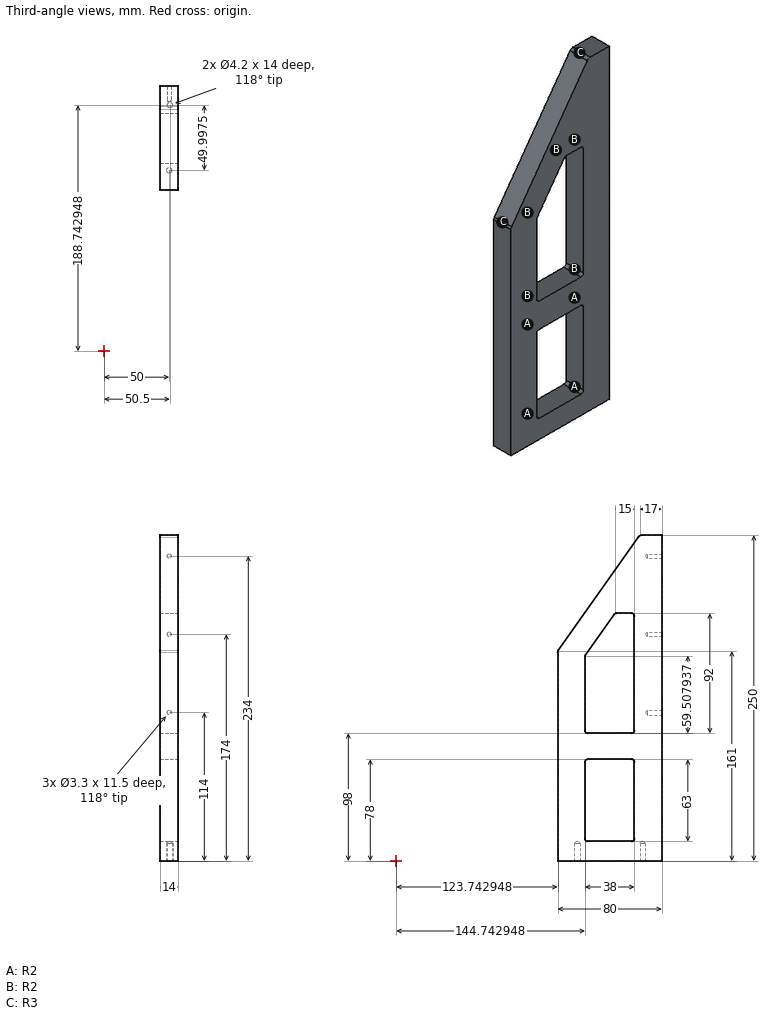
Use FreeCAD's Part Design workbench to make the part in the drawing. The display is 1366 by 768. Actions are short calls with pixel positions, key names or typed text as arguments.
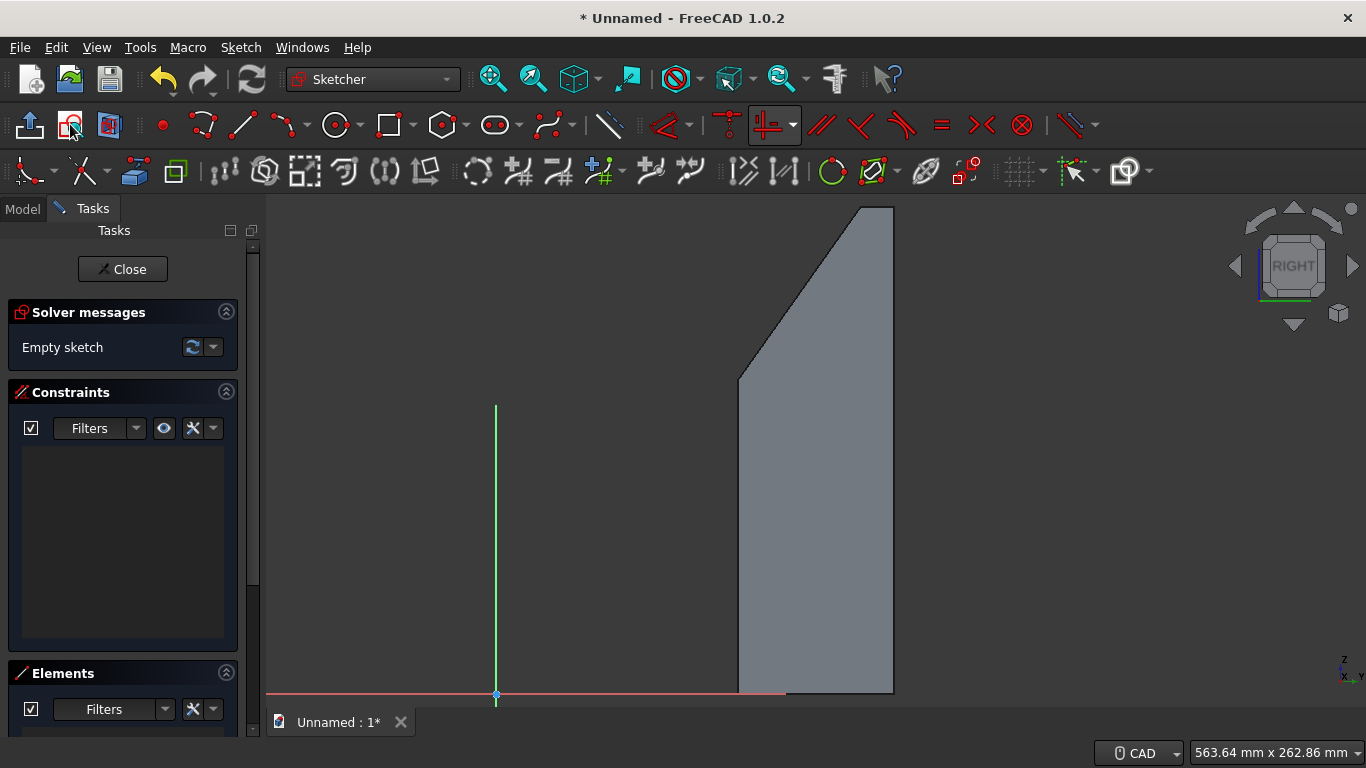
scroll(856, 679, up, 5)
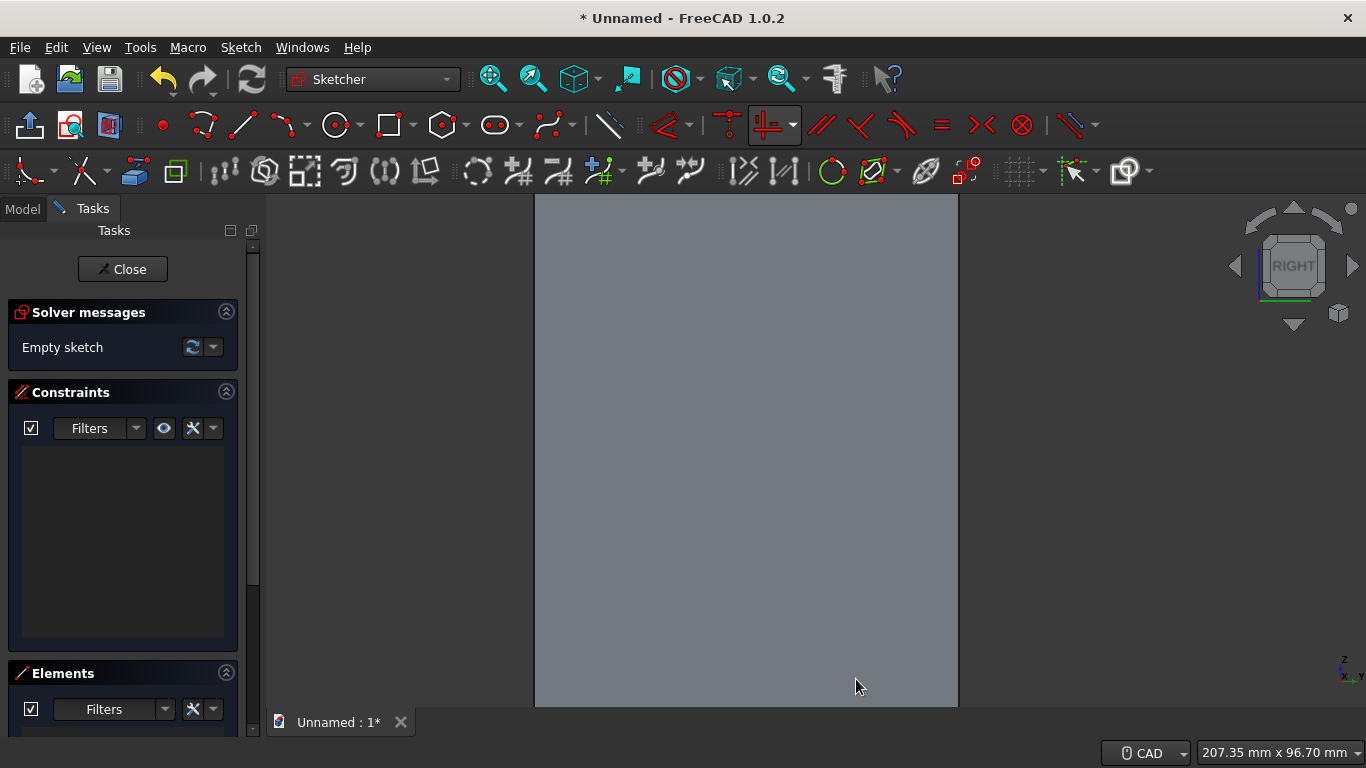
click(390, 126)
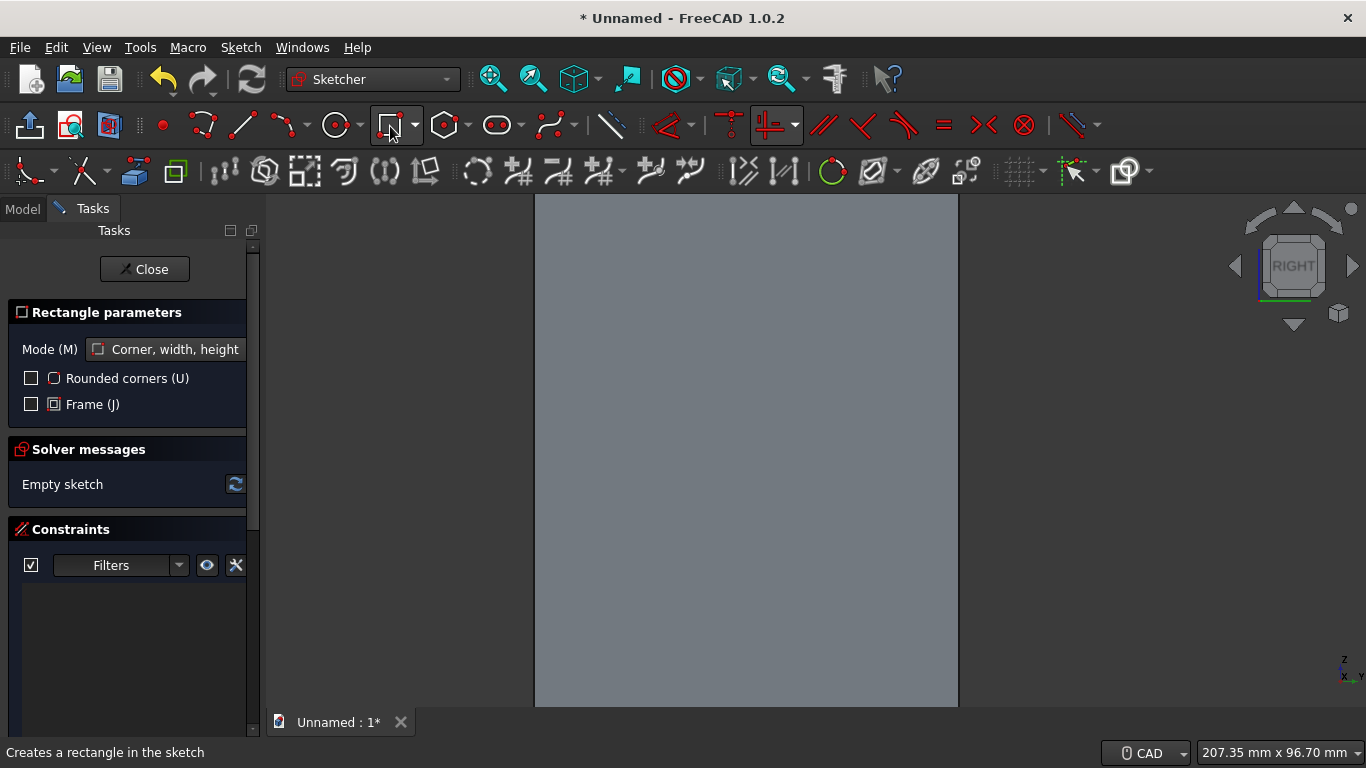
click(646, 306)
click(847, 640)
key(Escape)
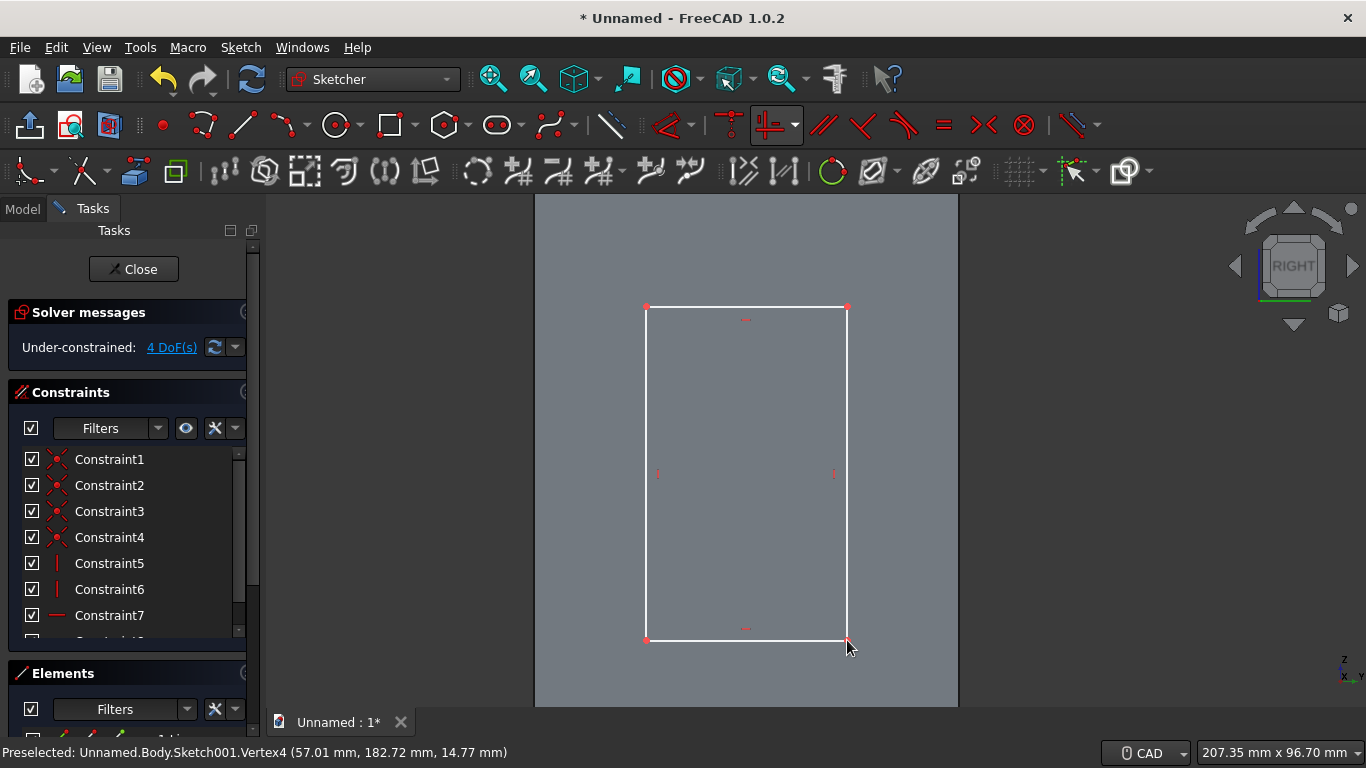
click(666, 126)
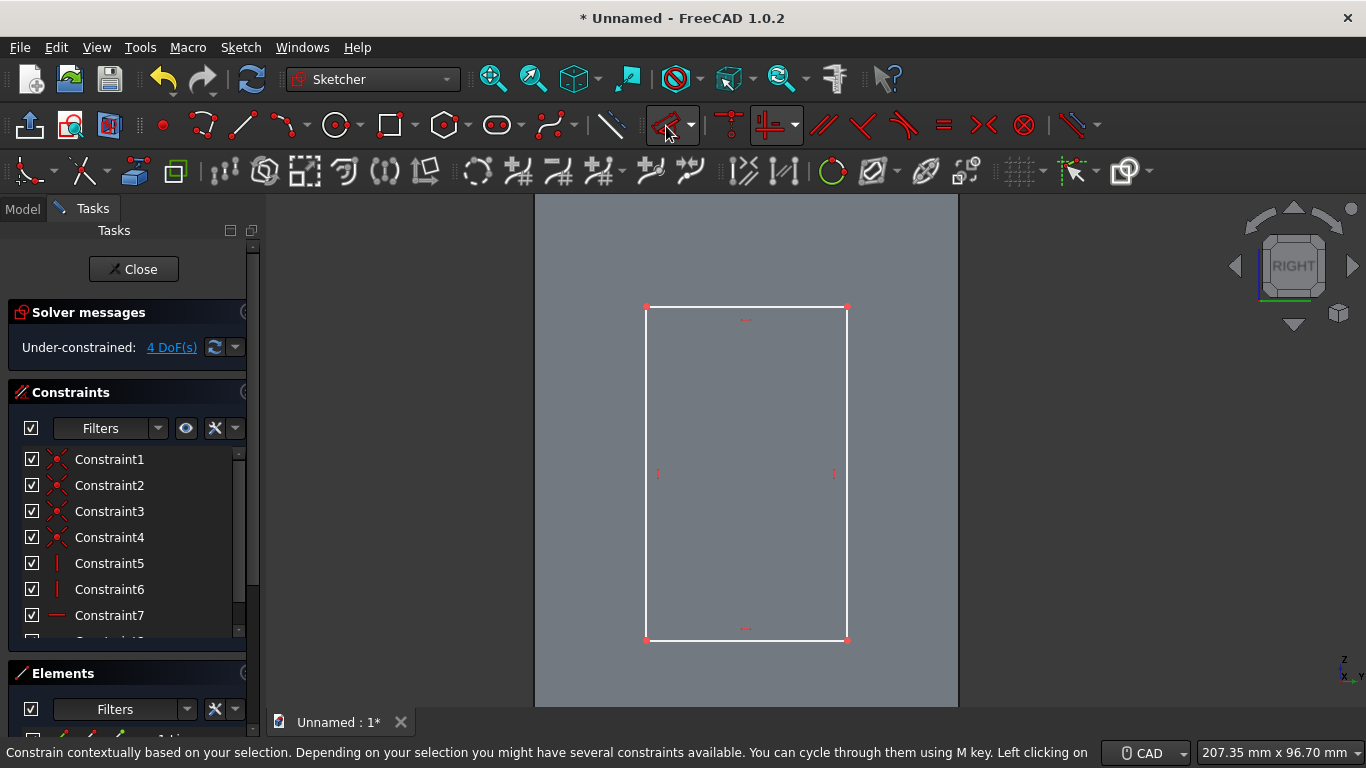
click(646, 407)
click(612, 474)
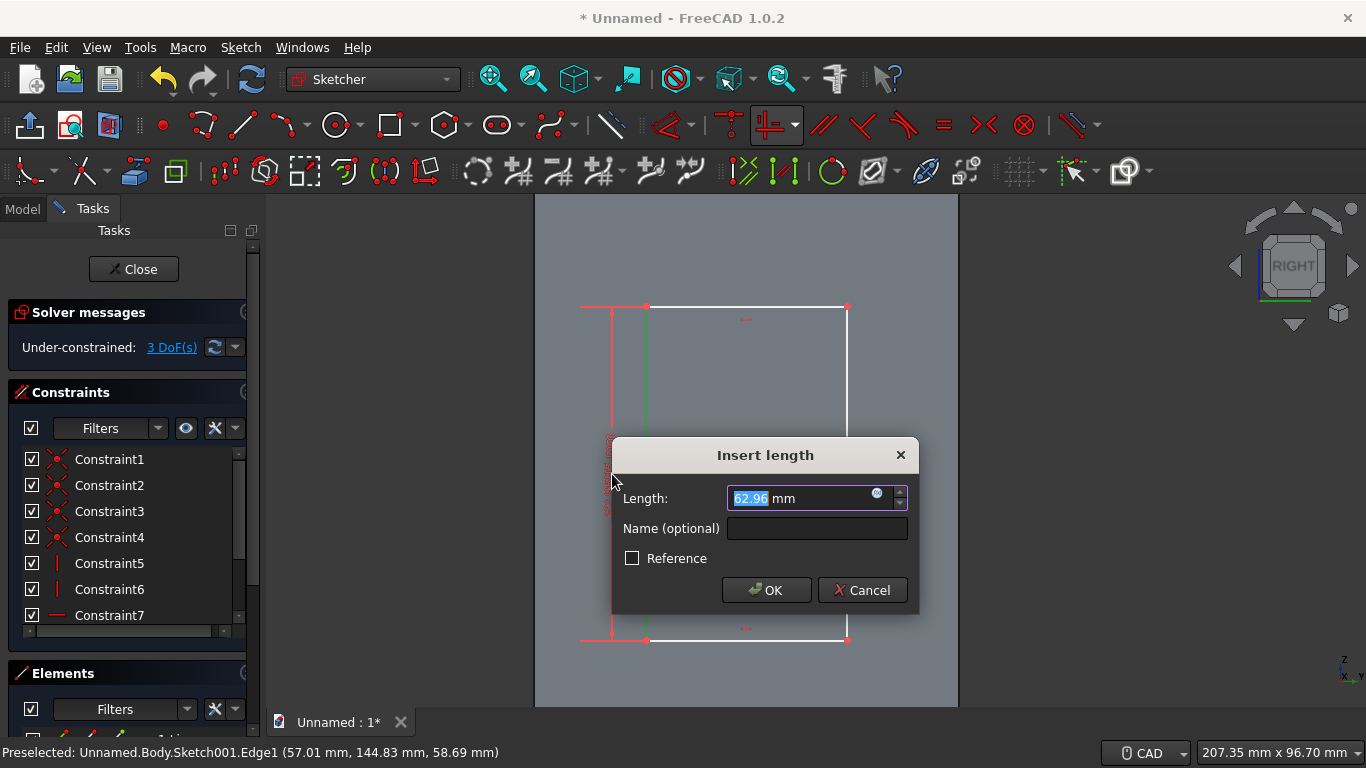
text(63)
key(Return)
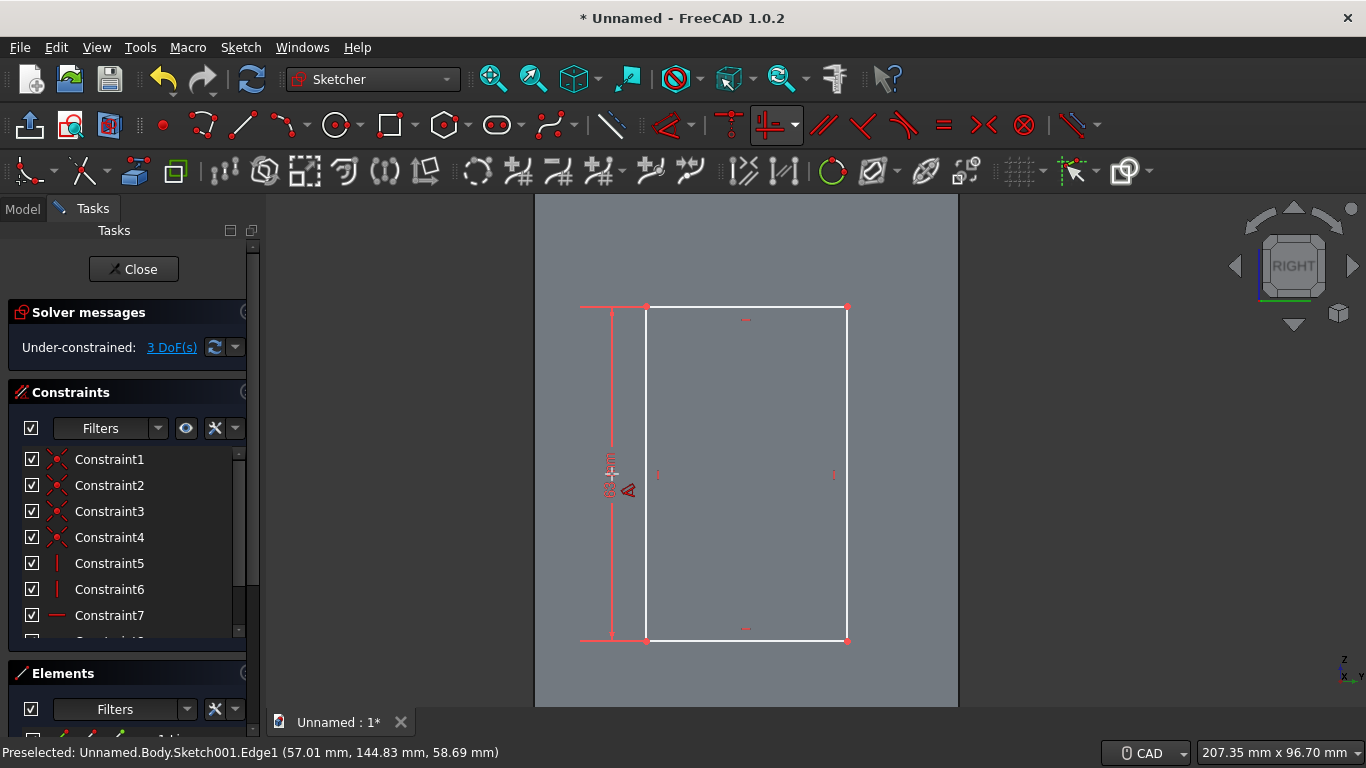
click(706, 641)
click(746, 675)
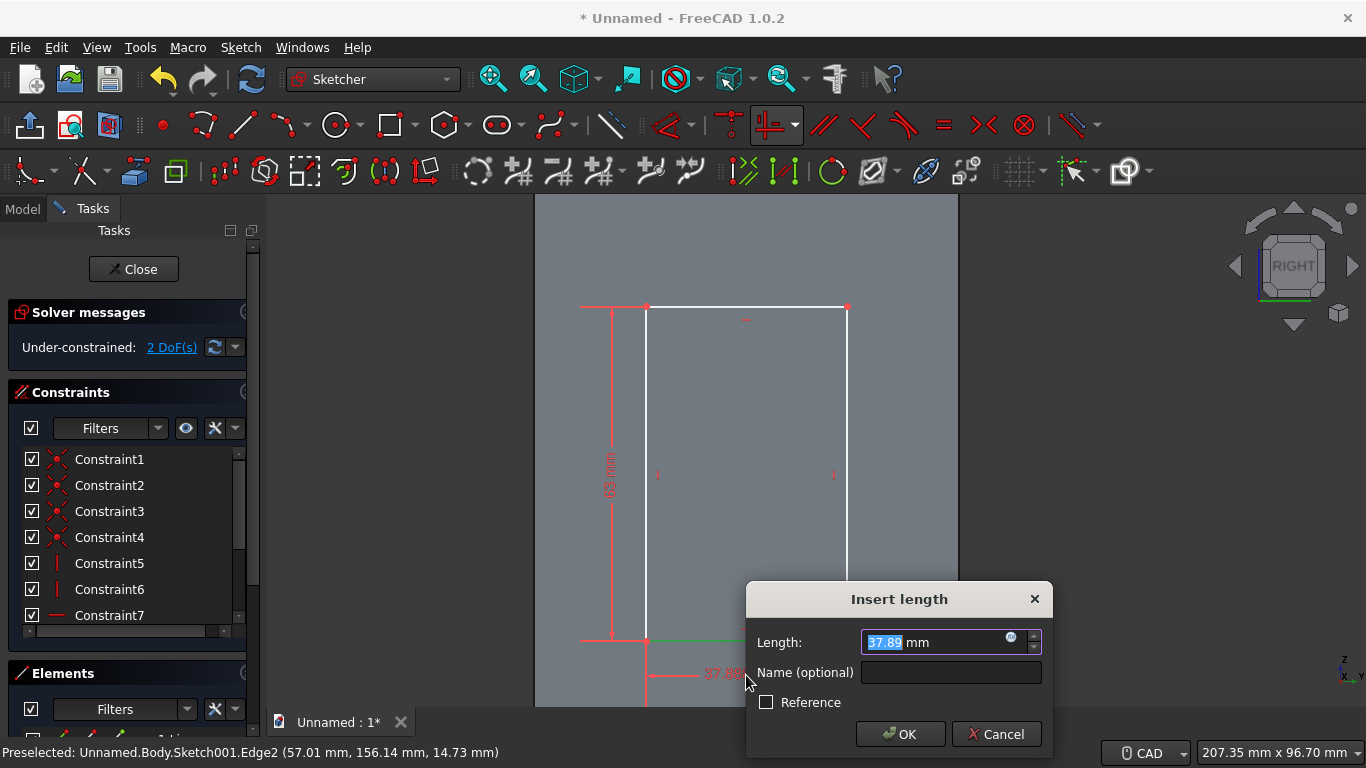
text(38)
key(Return)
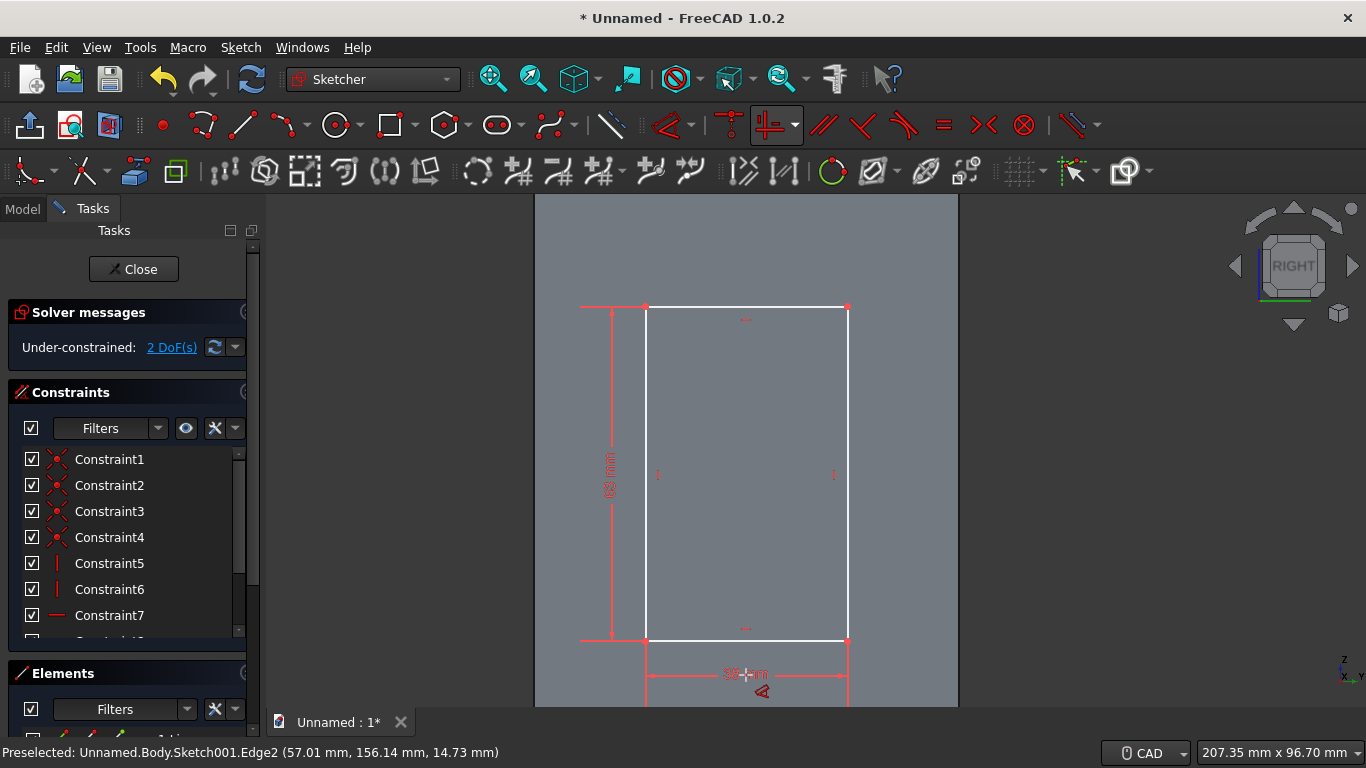
click(646, 307)
click(680, 407)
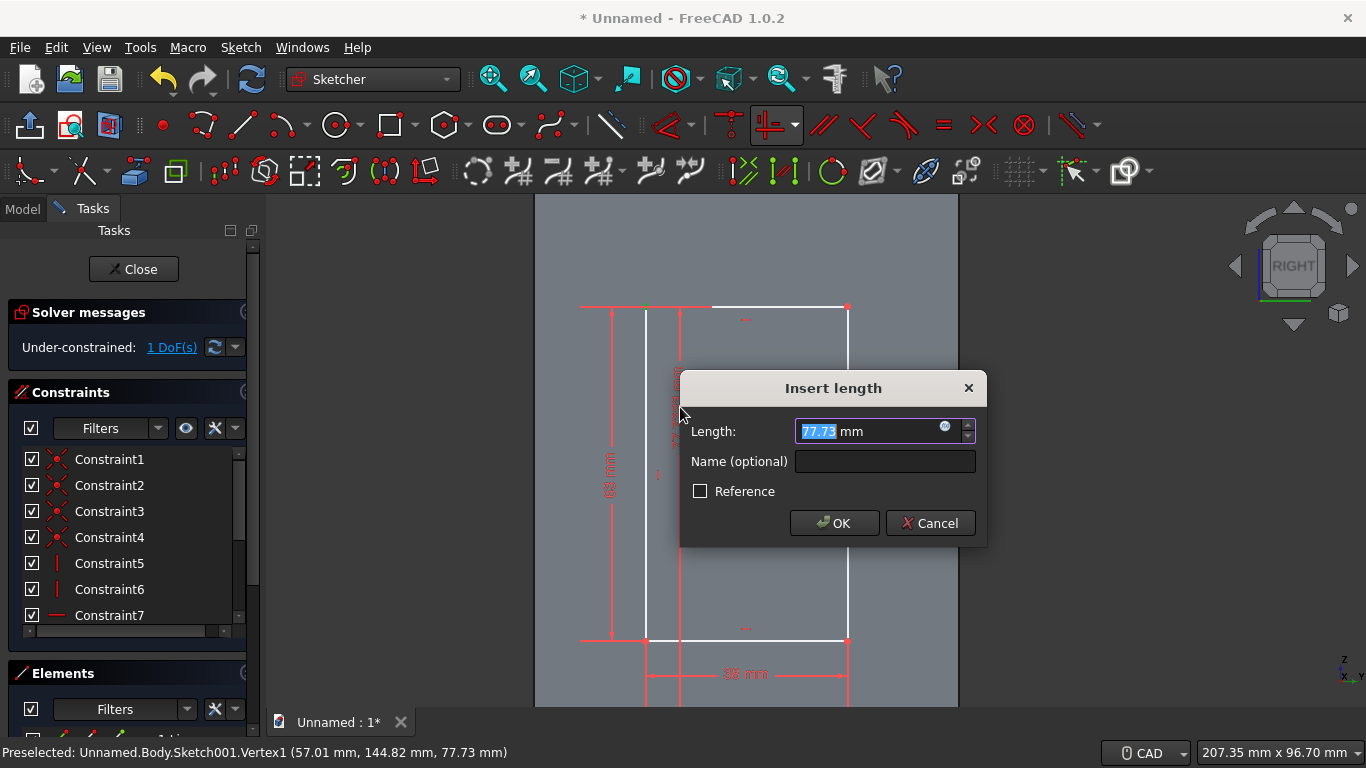
text(78)
key(Return)